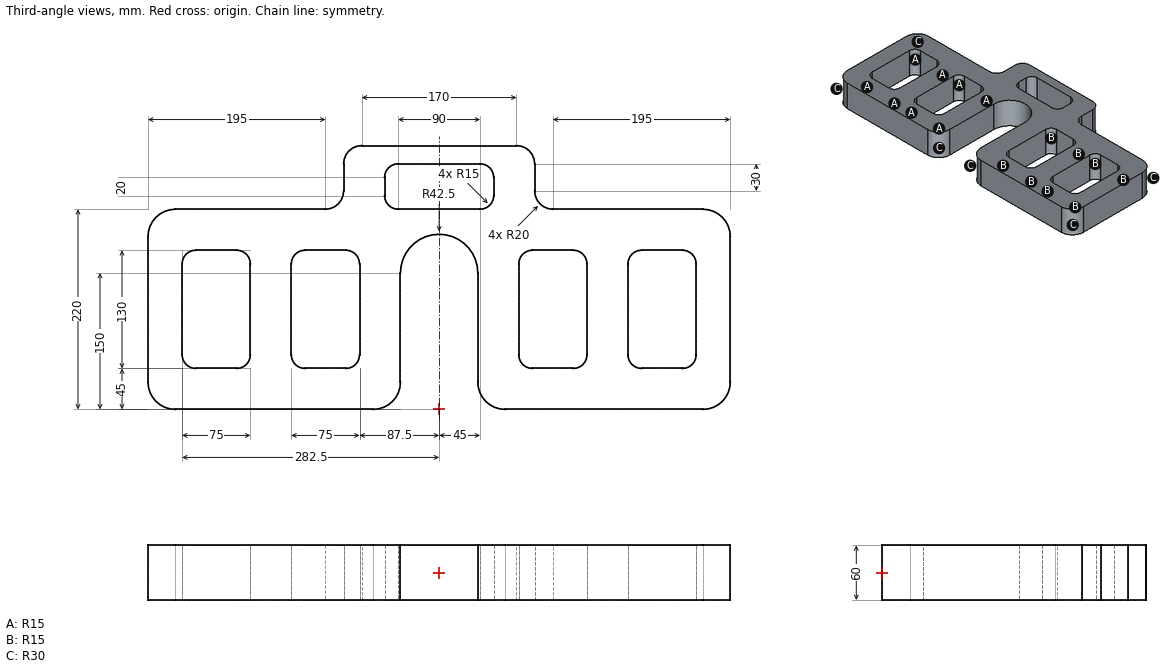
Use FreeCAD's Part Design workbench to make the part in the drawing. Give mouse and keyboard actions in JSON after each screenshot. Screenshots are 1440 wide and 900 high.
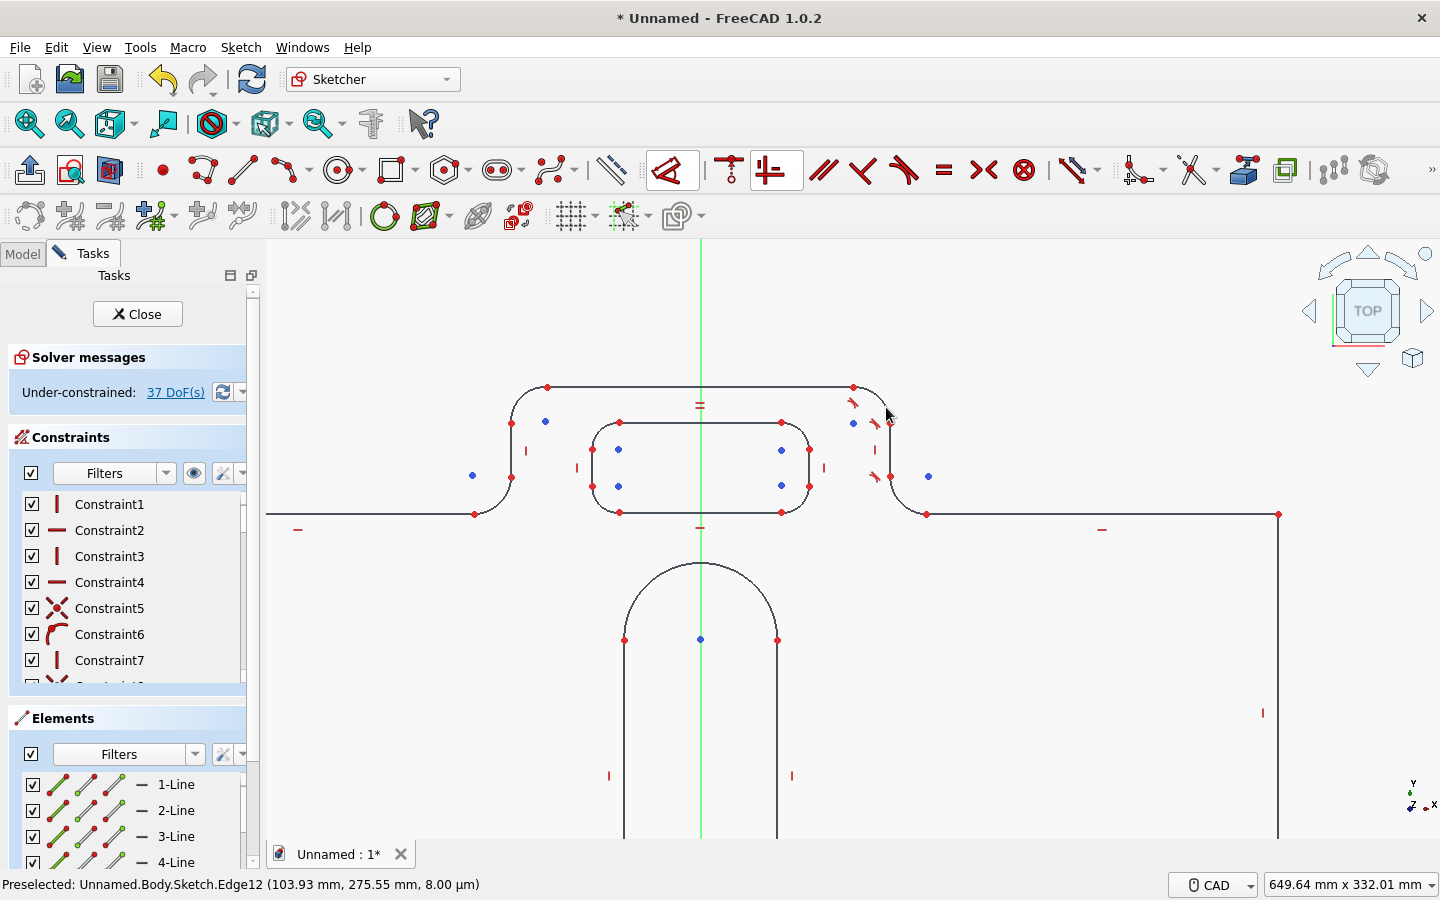
{"action": "left_click", "coordinate": [762, 387]}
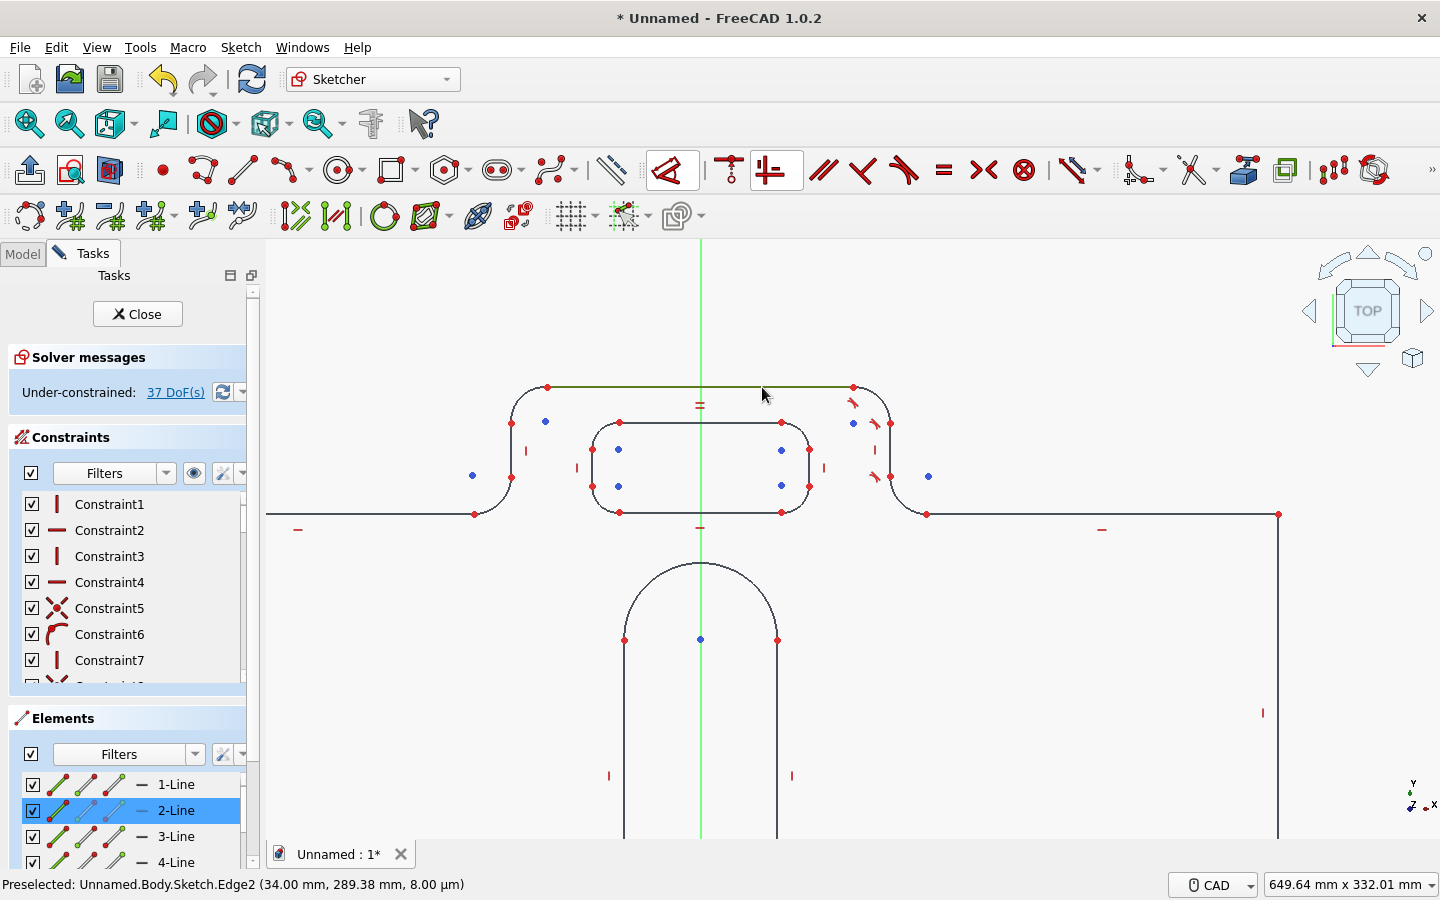
{"action": "left_click", "coordinate": [531, 390]}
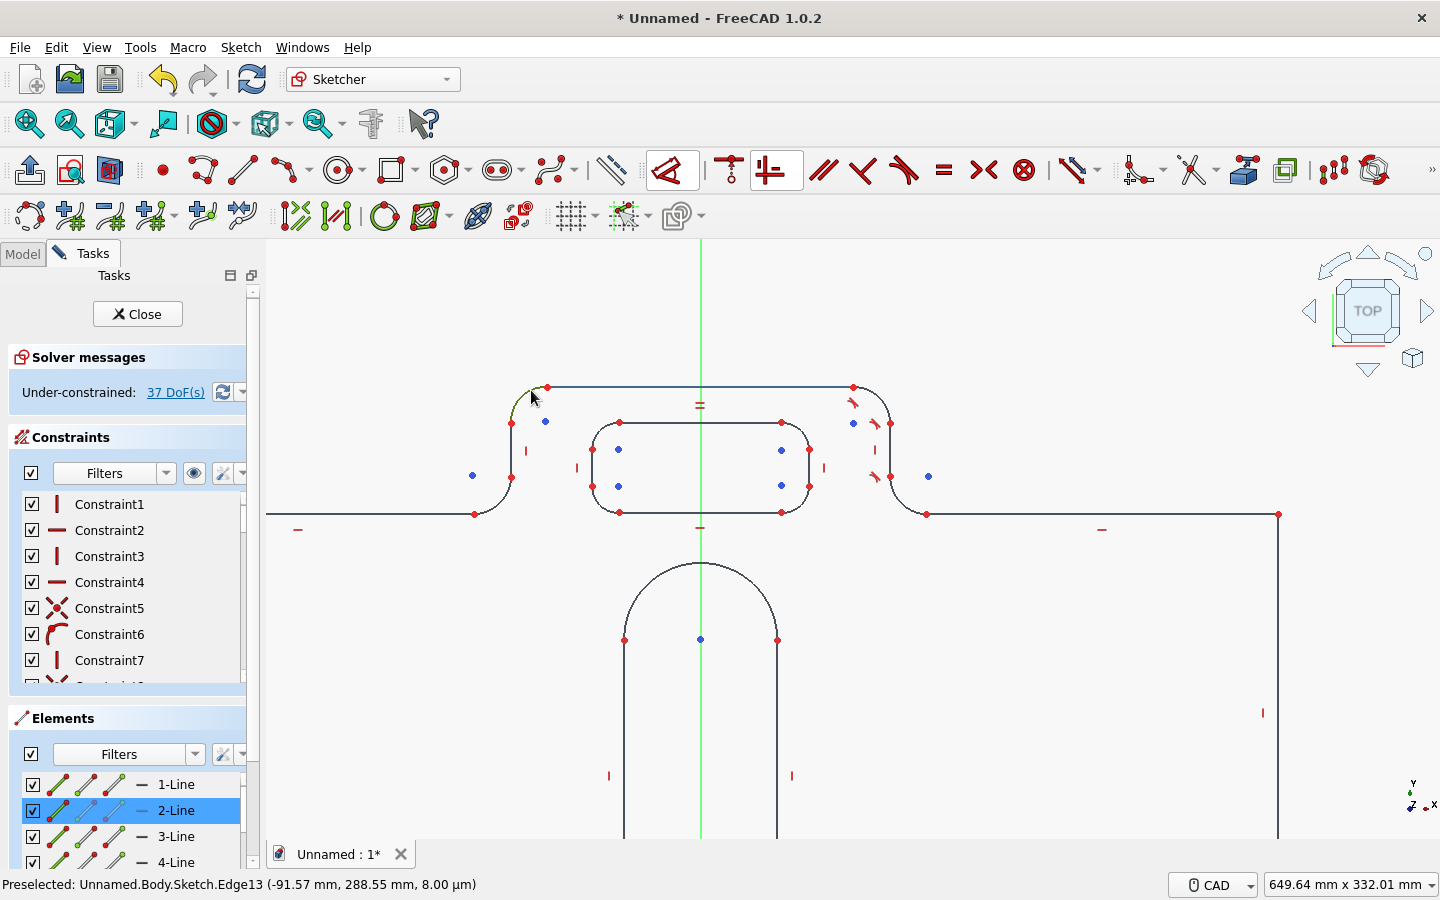
{"action": "left_click", "coordinate": [904, 170]}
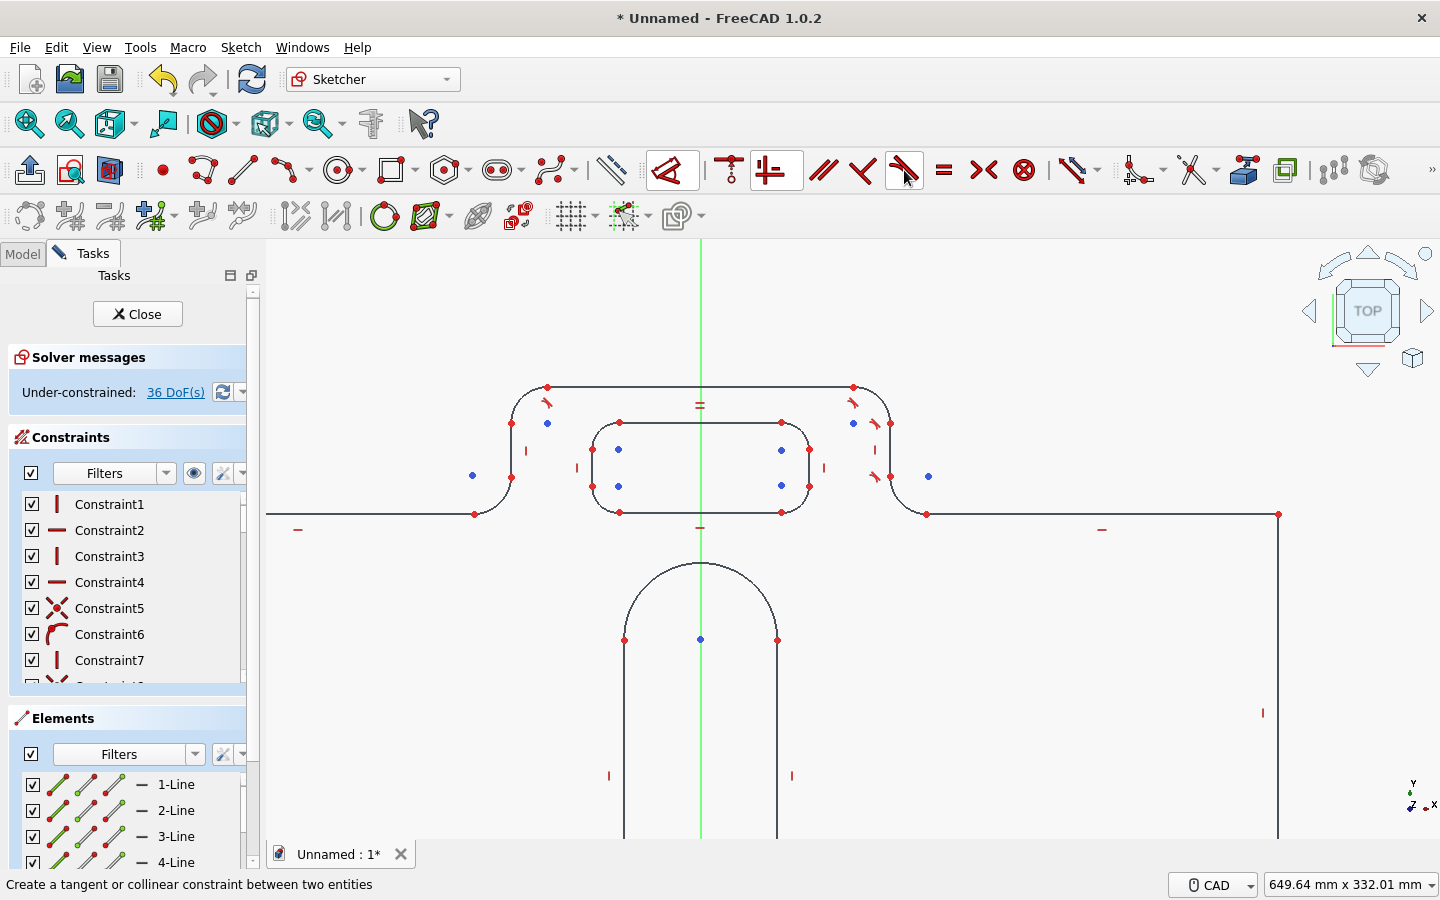
{"action": "left_click", "coordinate": [511, 440]}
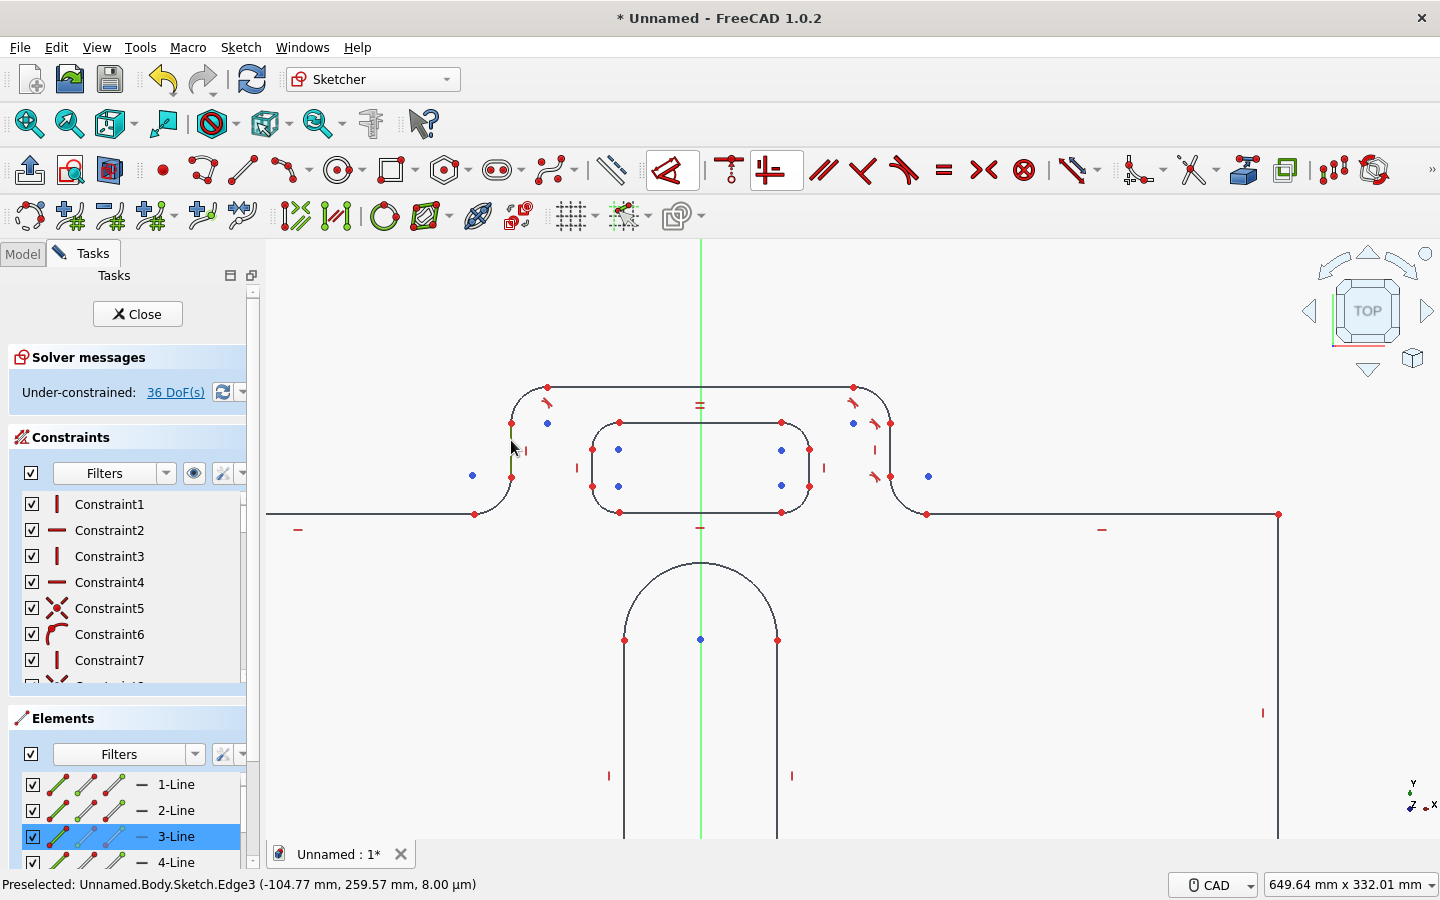
{"action": "left_click", "coordinate": [531, 391]}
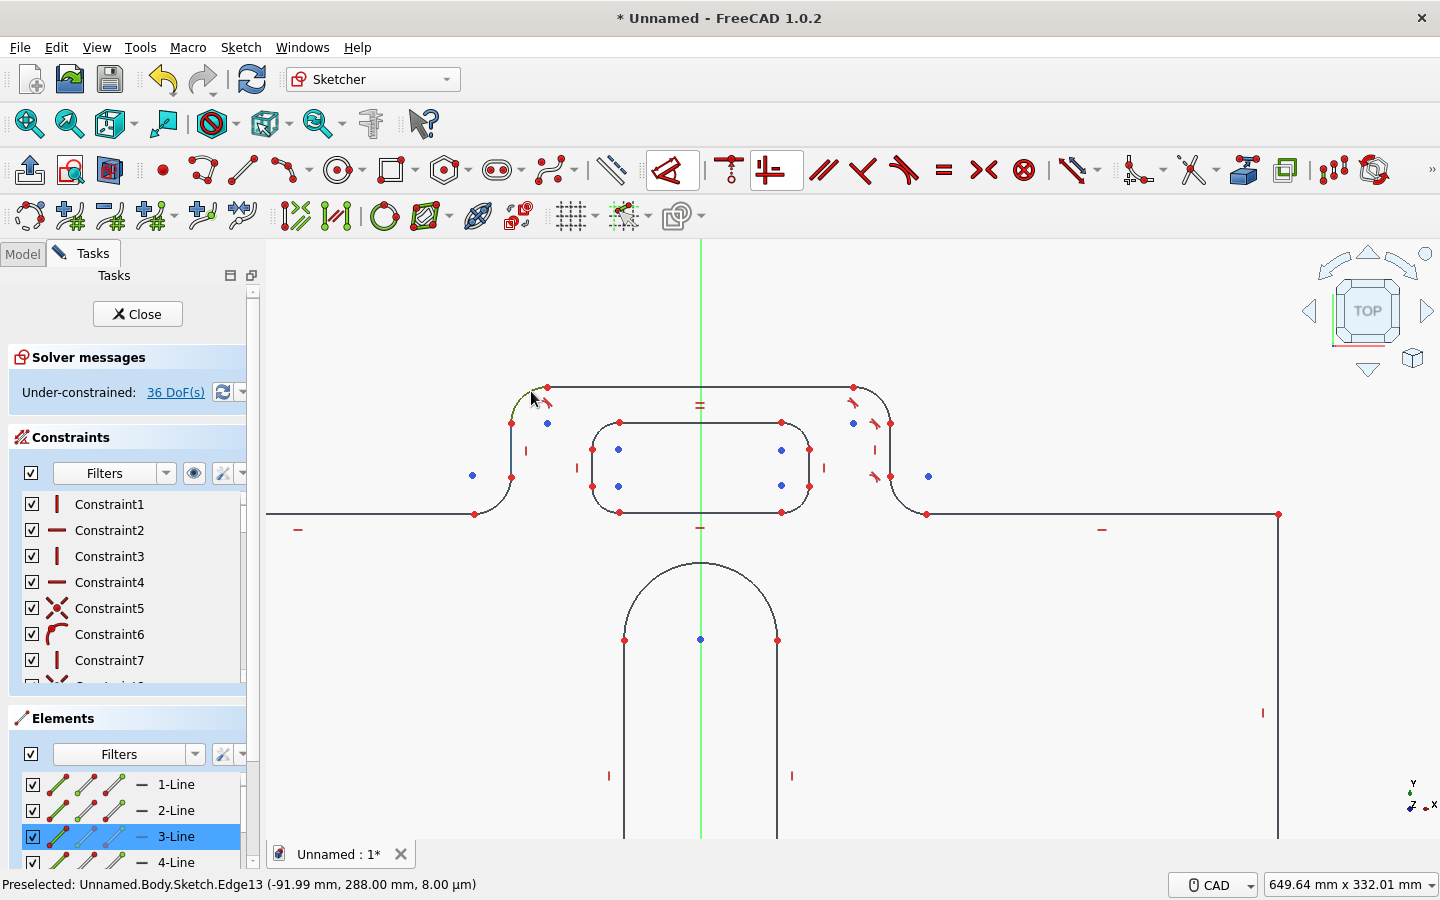
{"action": "left_click", "coordinate": [904, 170]}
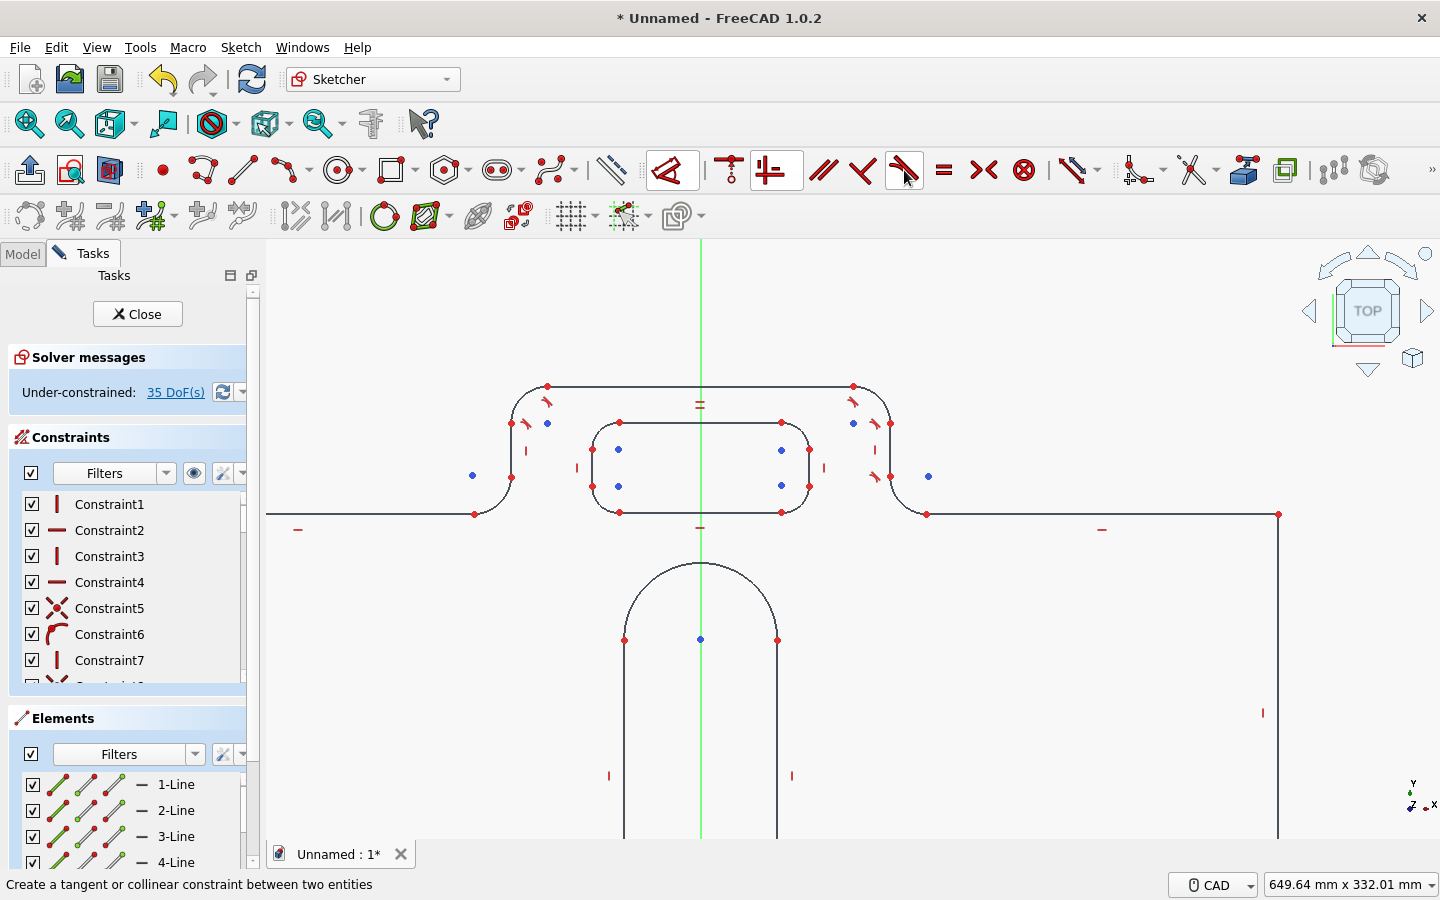
{"action": "left_click", "coordinate": [511, 440]}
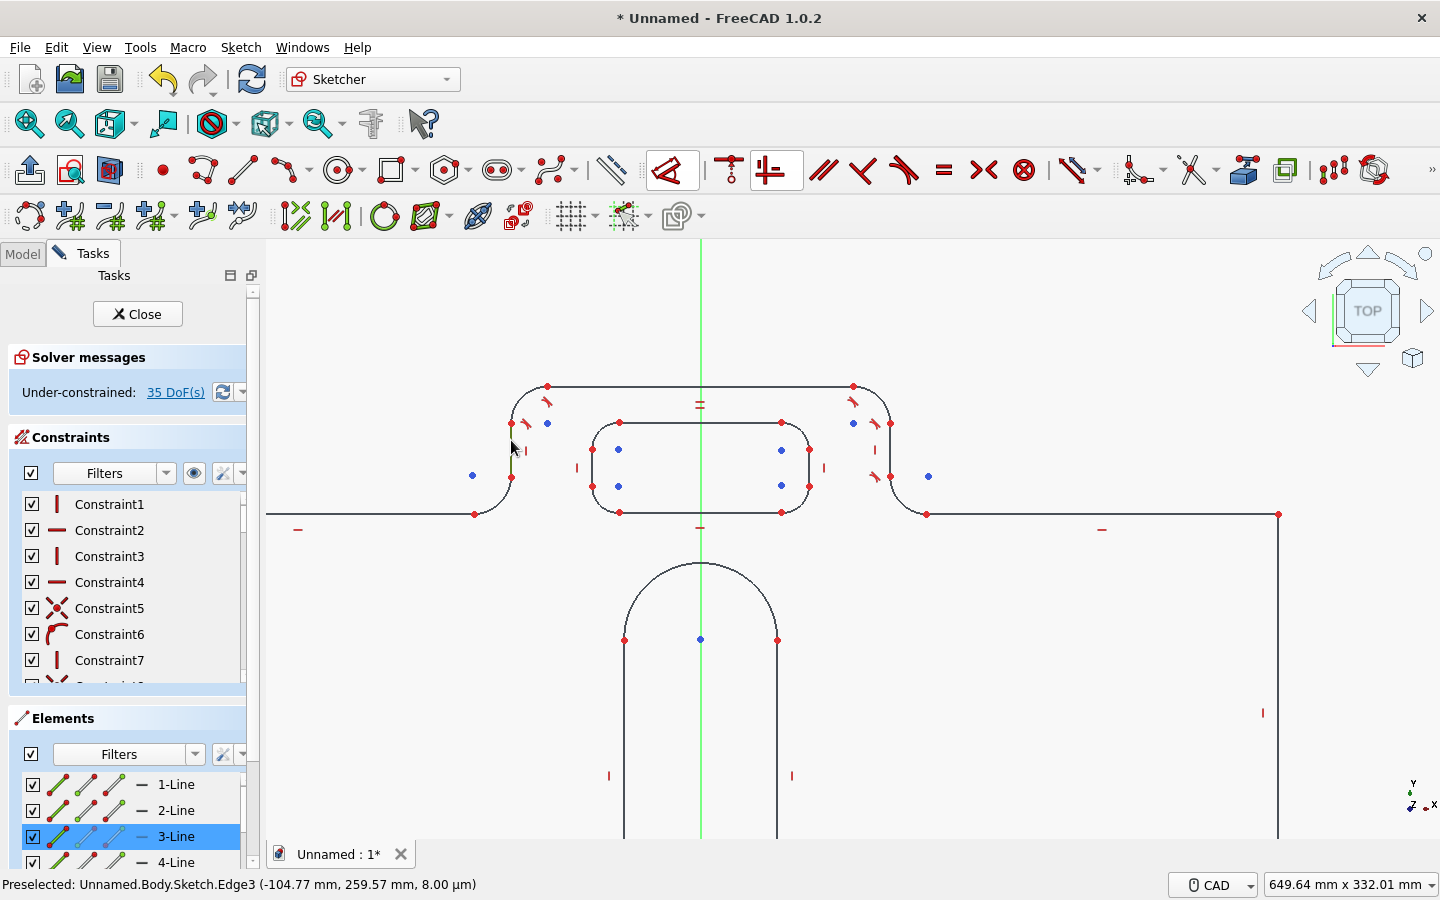
{"action": "left_click", "coordinate": [491, 510]}